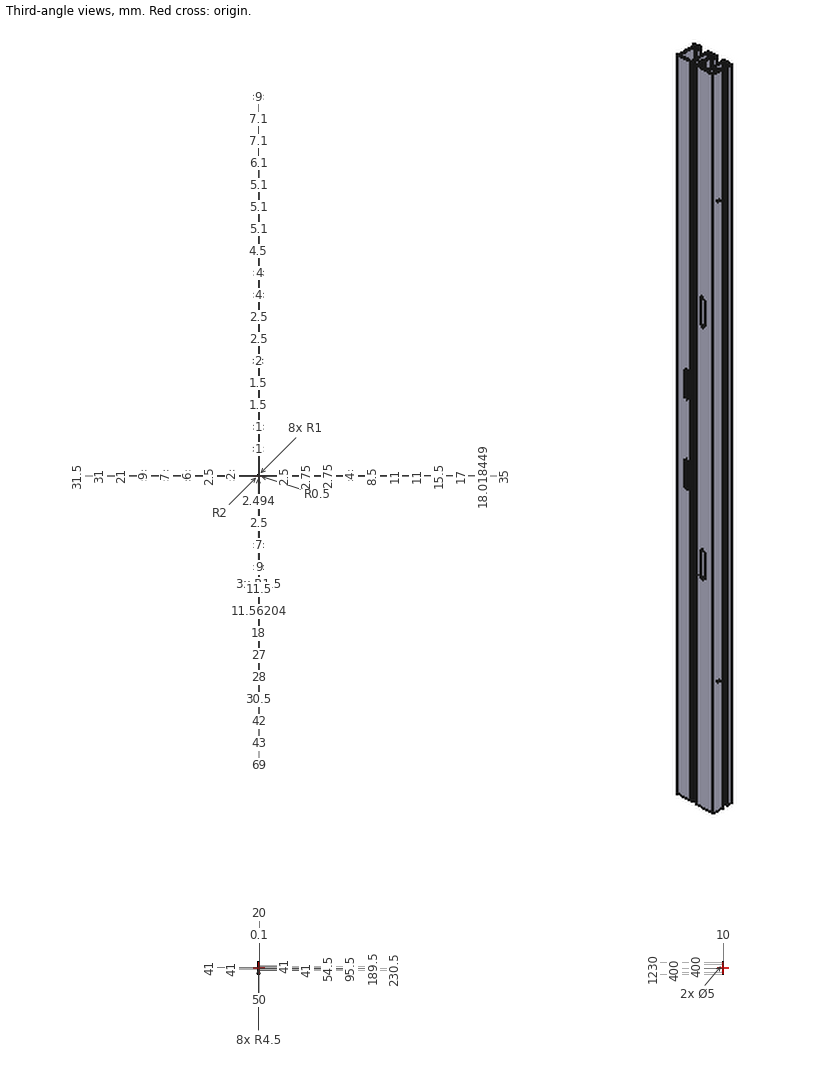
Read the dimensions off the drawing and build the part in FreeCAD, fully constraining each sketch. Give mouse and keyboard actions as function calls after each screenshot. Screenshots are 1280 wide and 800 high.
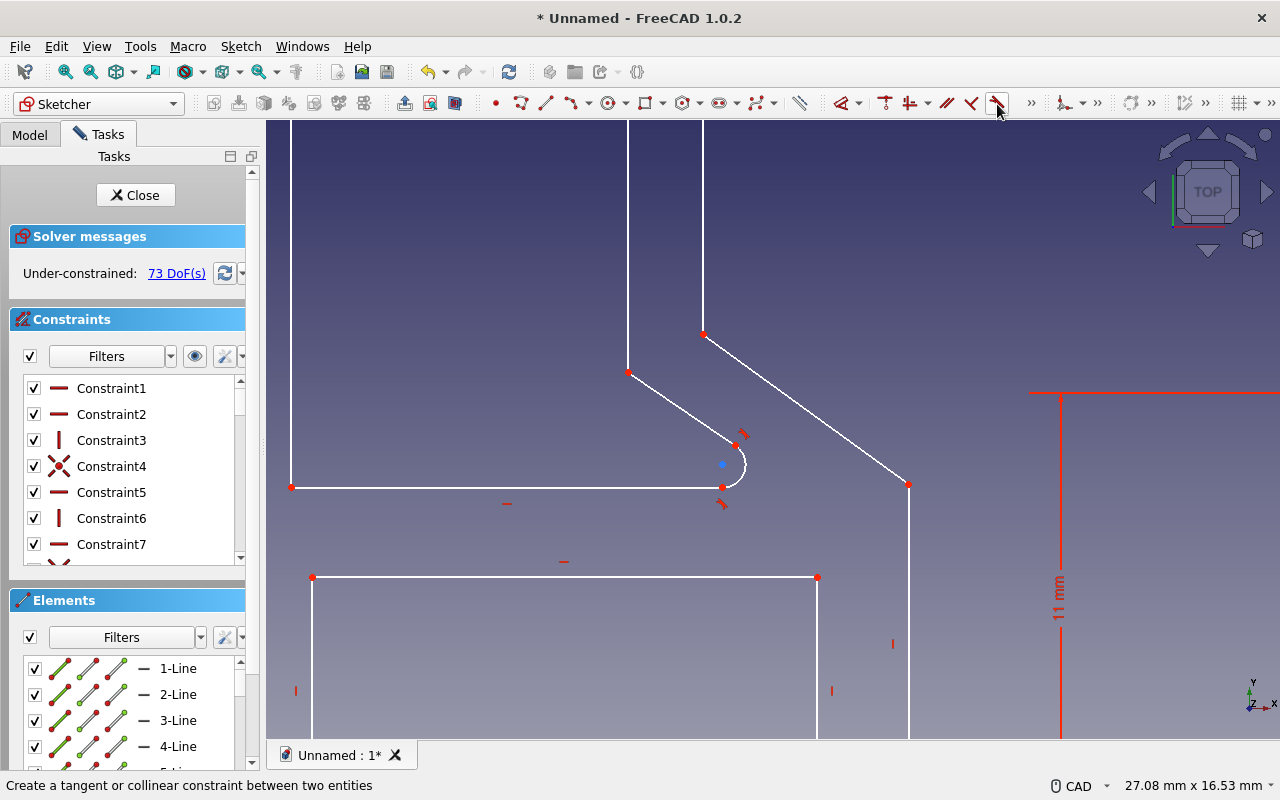
scroll(742, 478, down, 8)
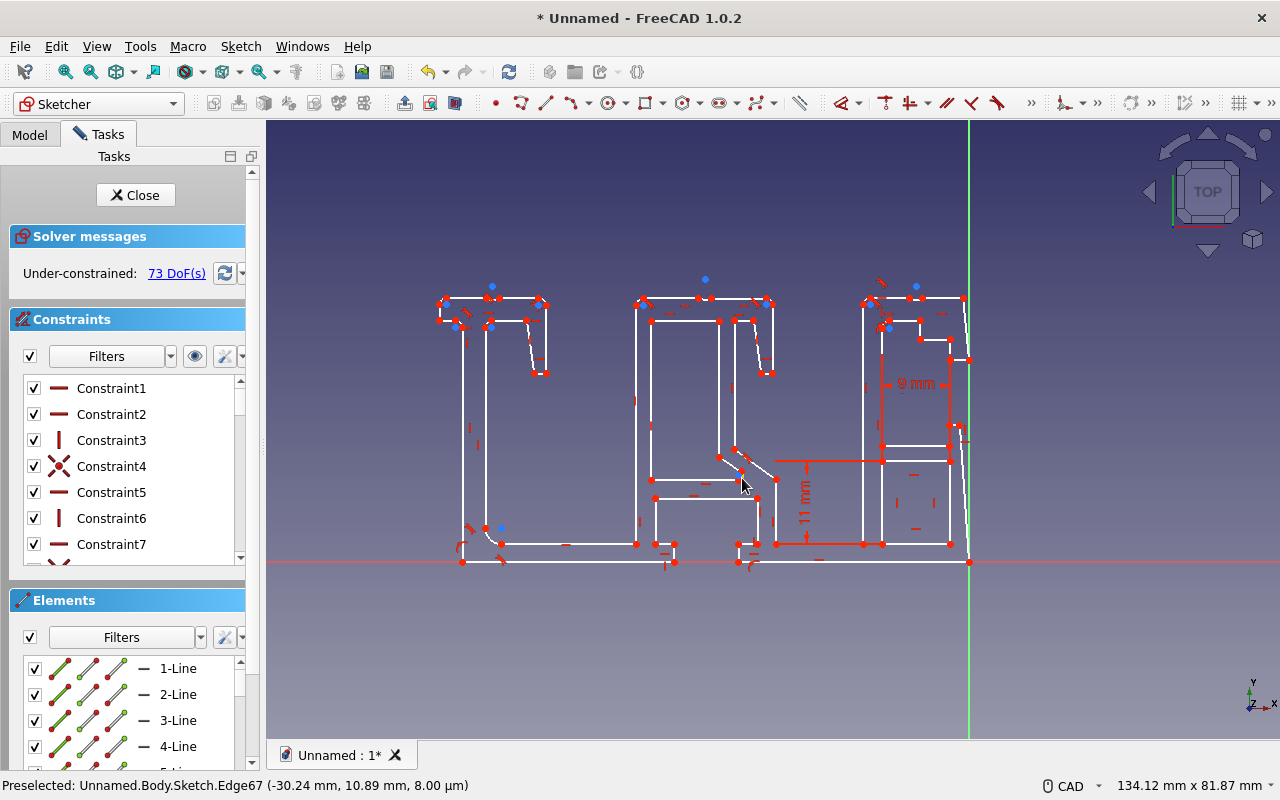
scroll(966, 521, up, 8)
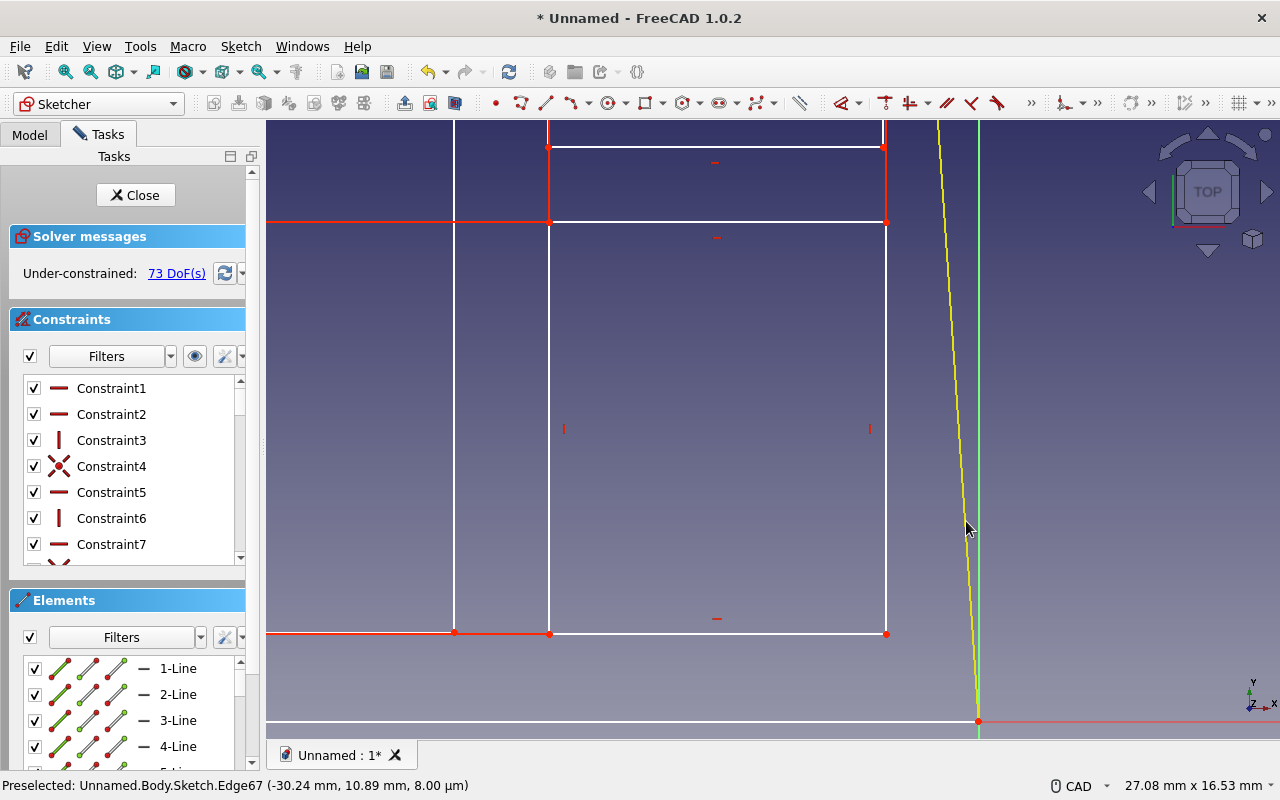
click(965, 518)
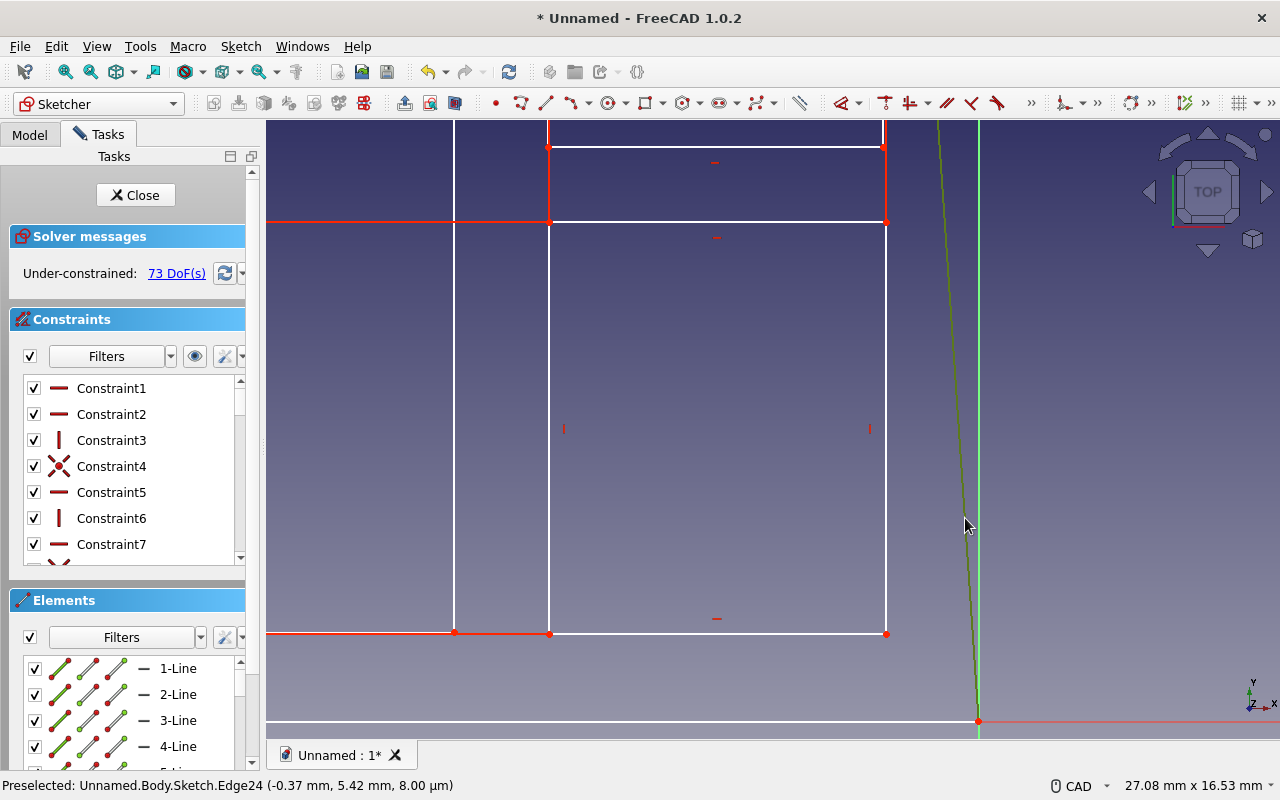
click(928, 104)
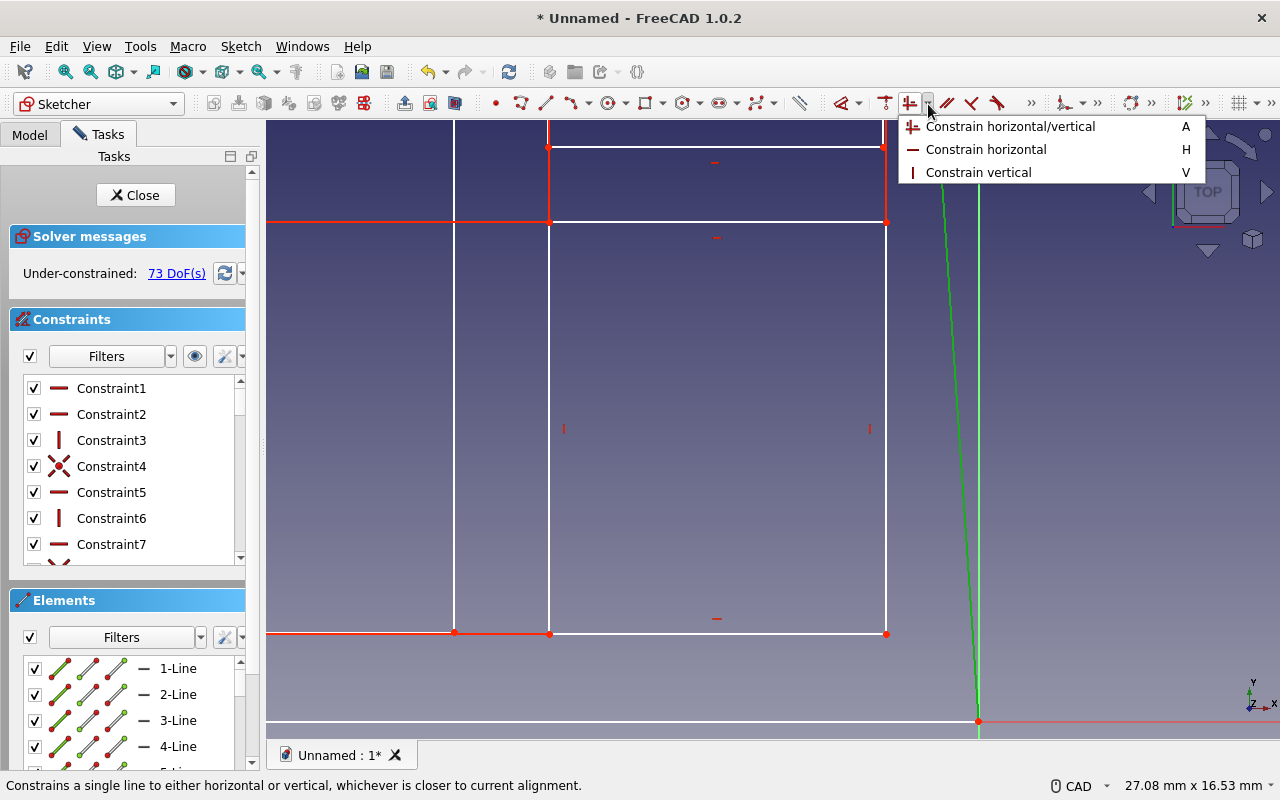
click(1052, 172)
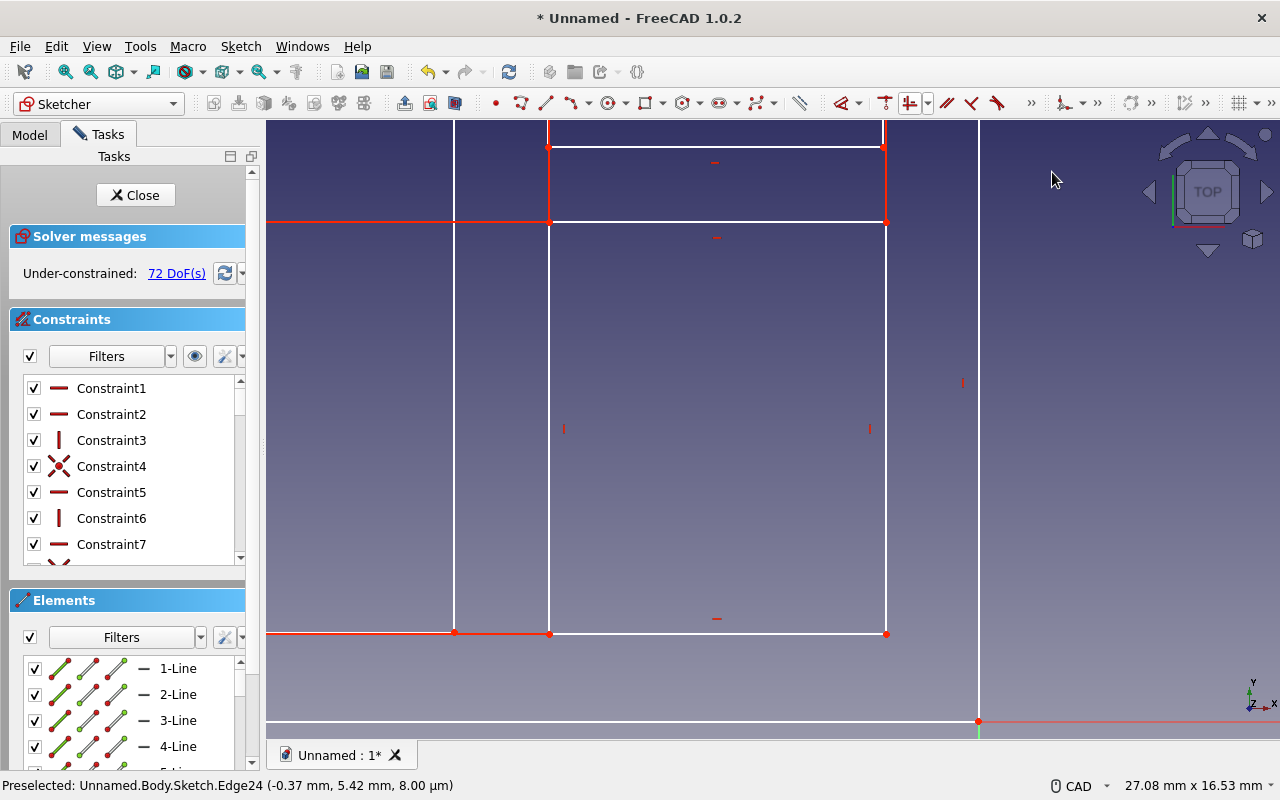
scroll(967, 521, down, 8)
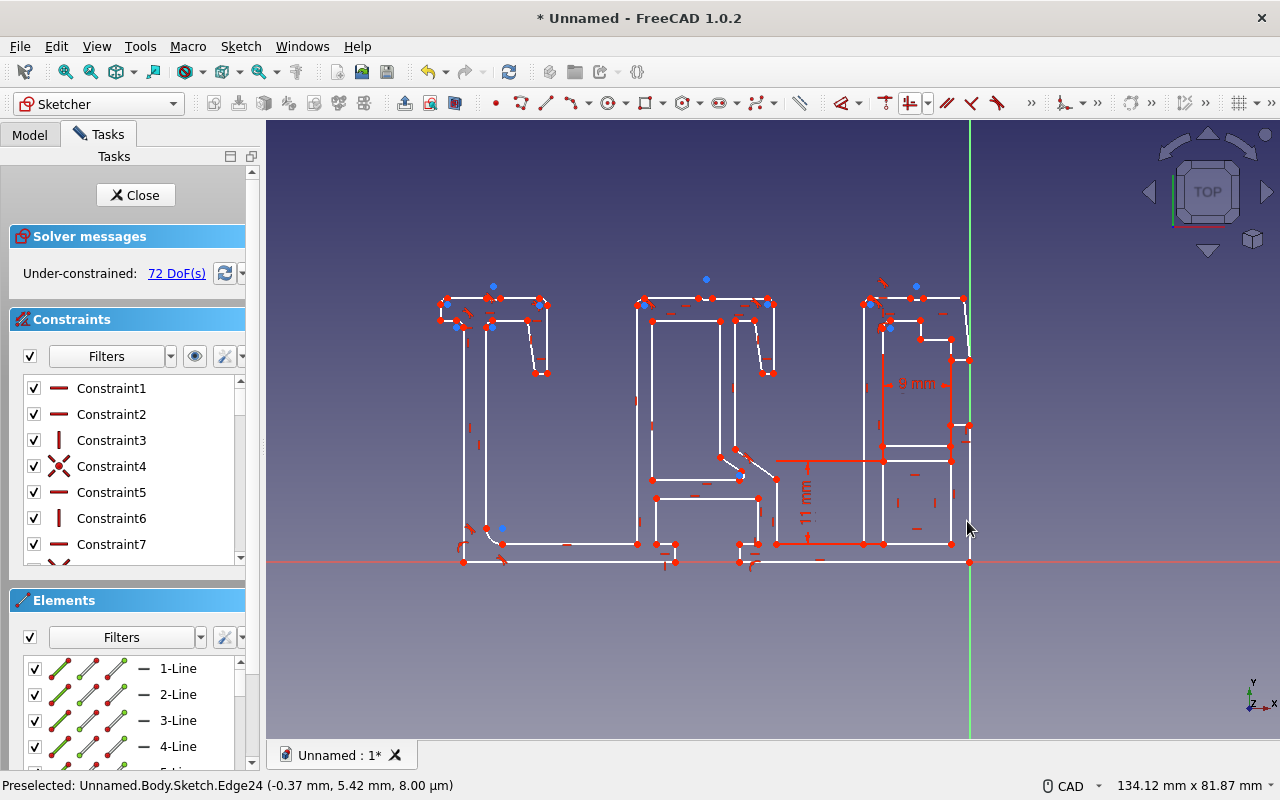
scroll(966, 317, up, 6)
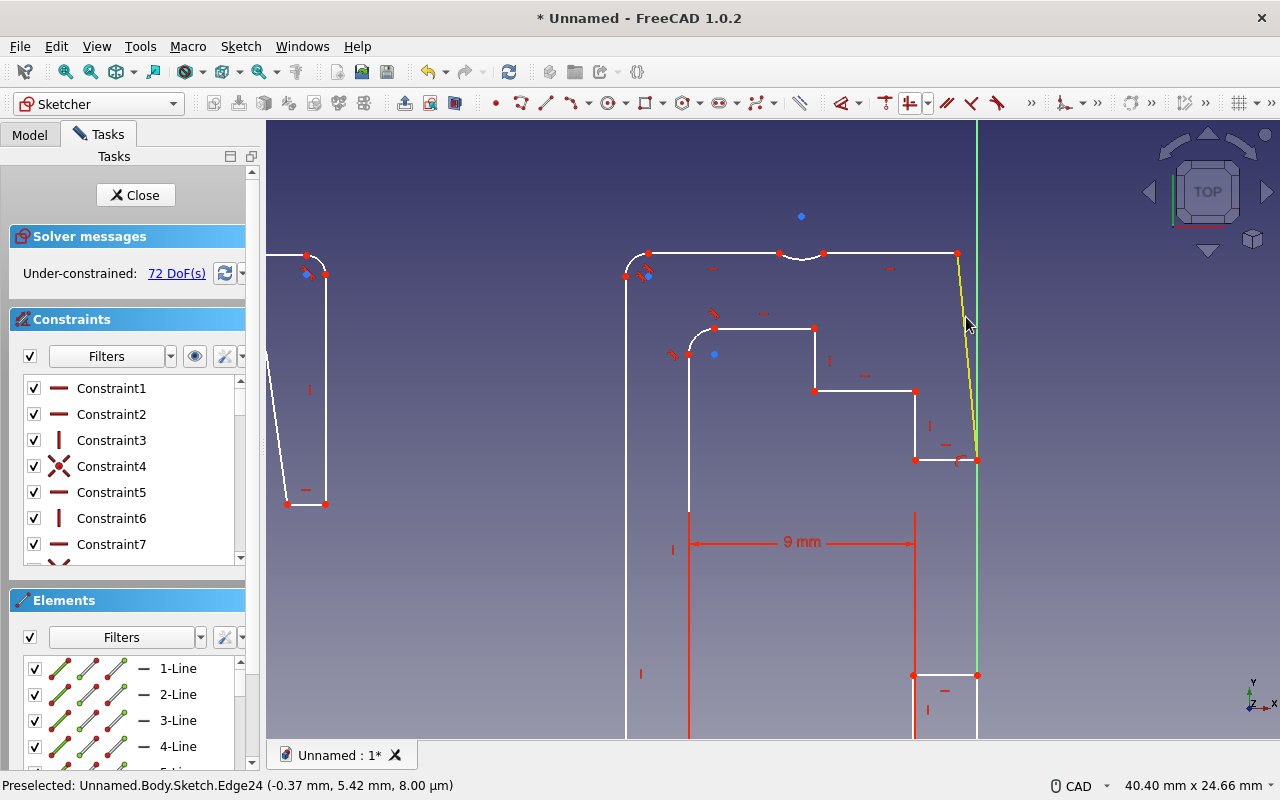
click(963, 316)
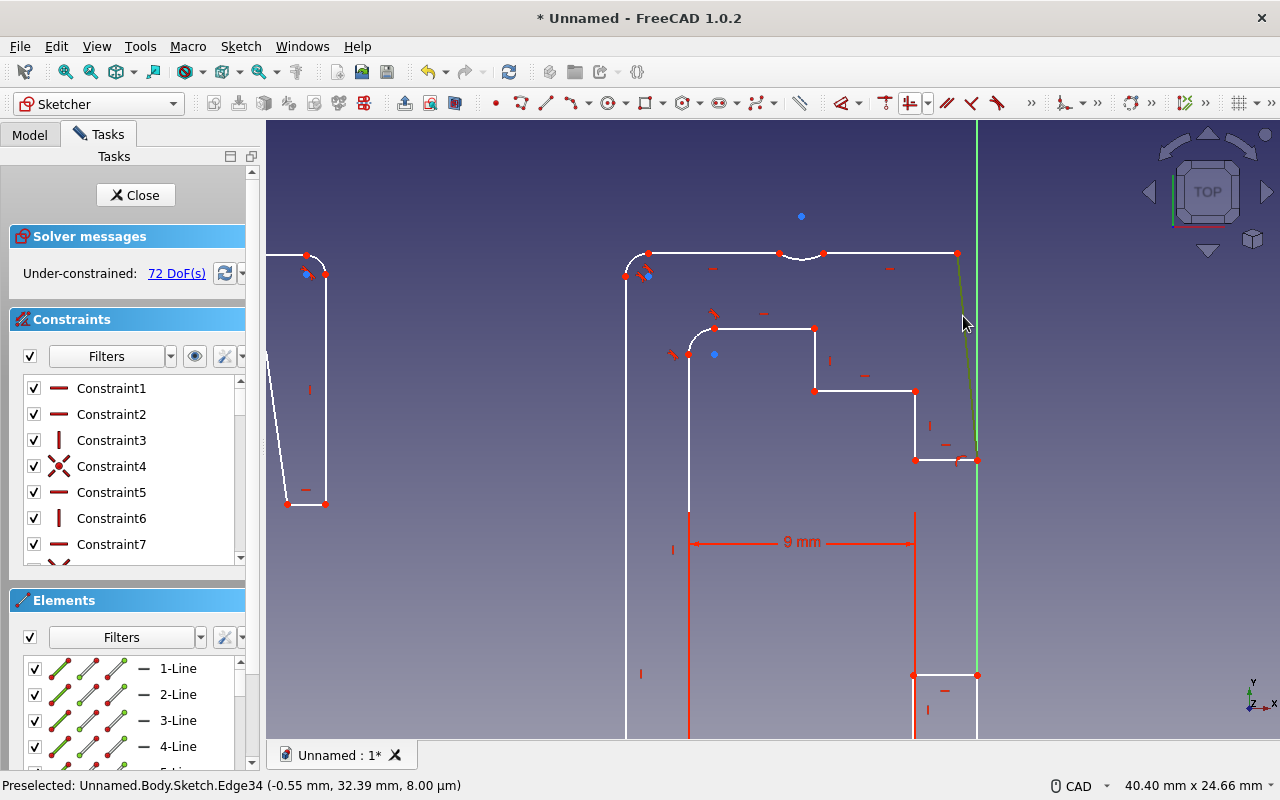
click(928, 104)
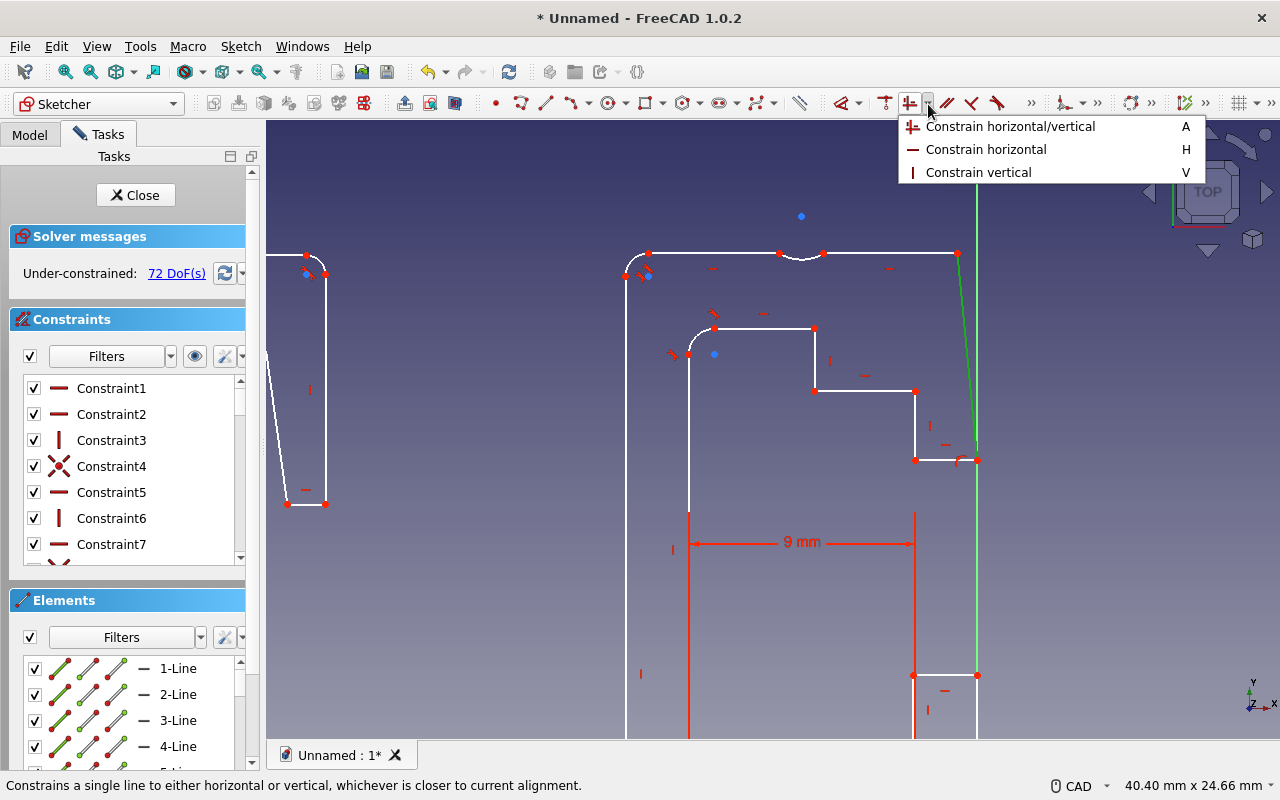
click(1052, 172)